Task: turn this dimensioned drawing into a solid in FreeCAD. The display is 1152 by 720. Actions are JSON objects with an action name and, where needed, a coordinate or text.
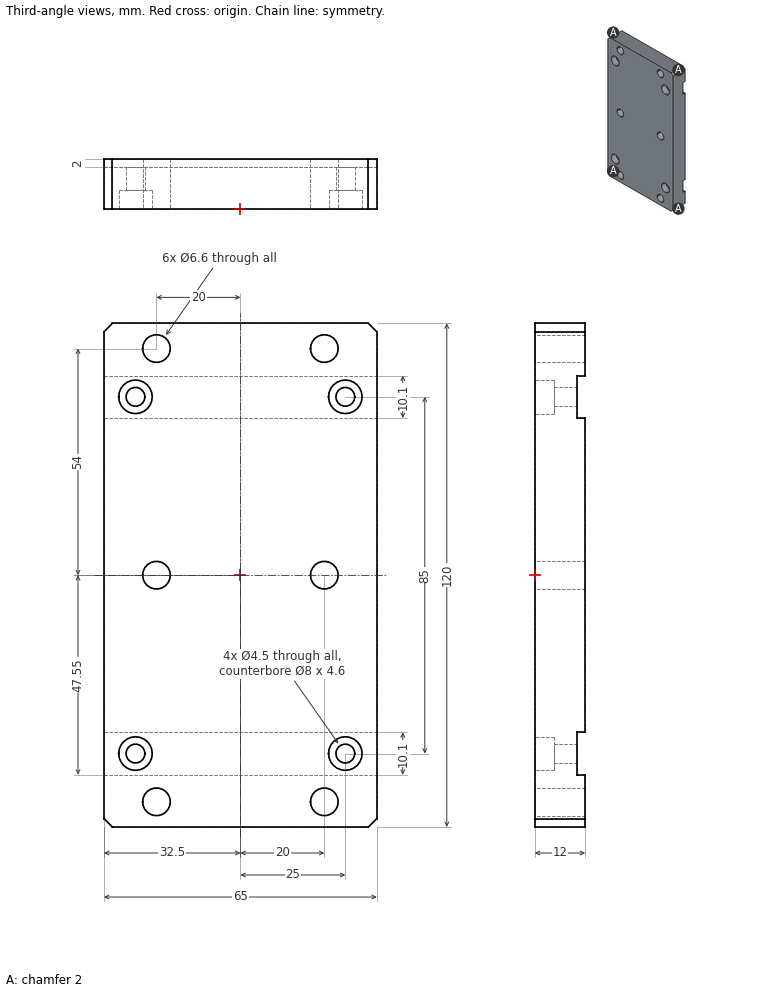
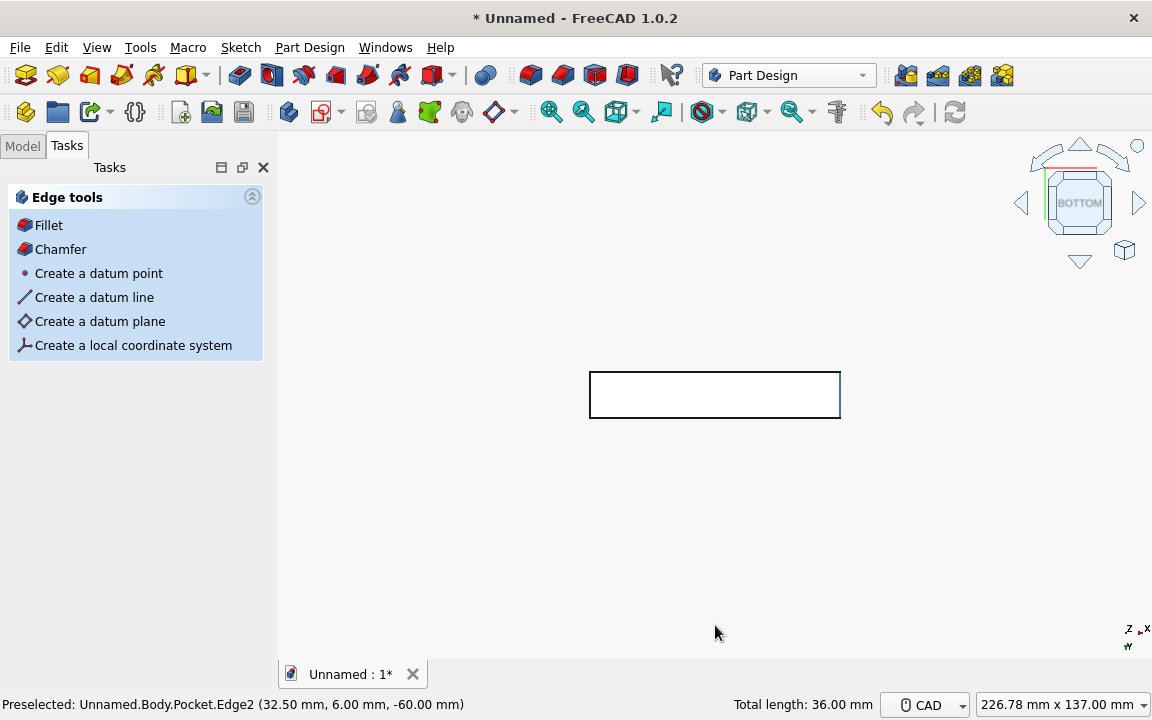
{"action": "key", "text": "v f"}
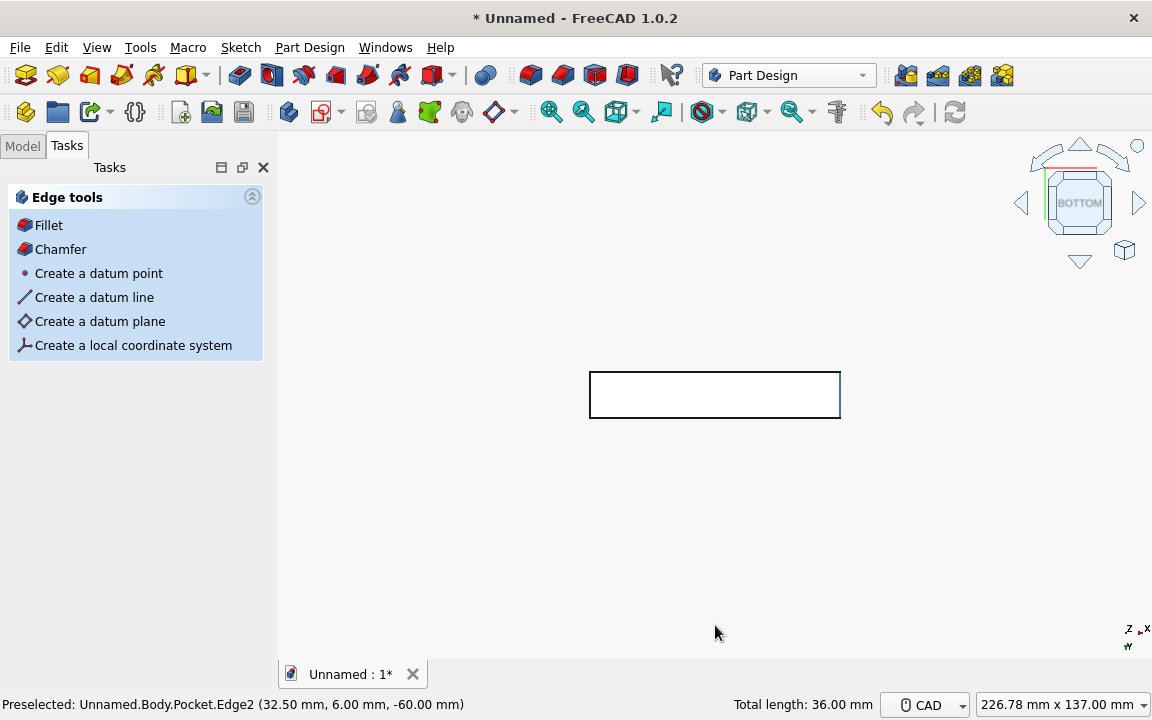
{"action": "left_click", "coordinate": [590, 394], "text": "ctrl"}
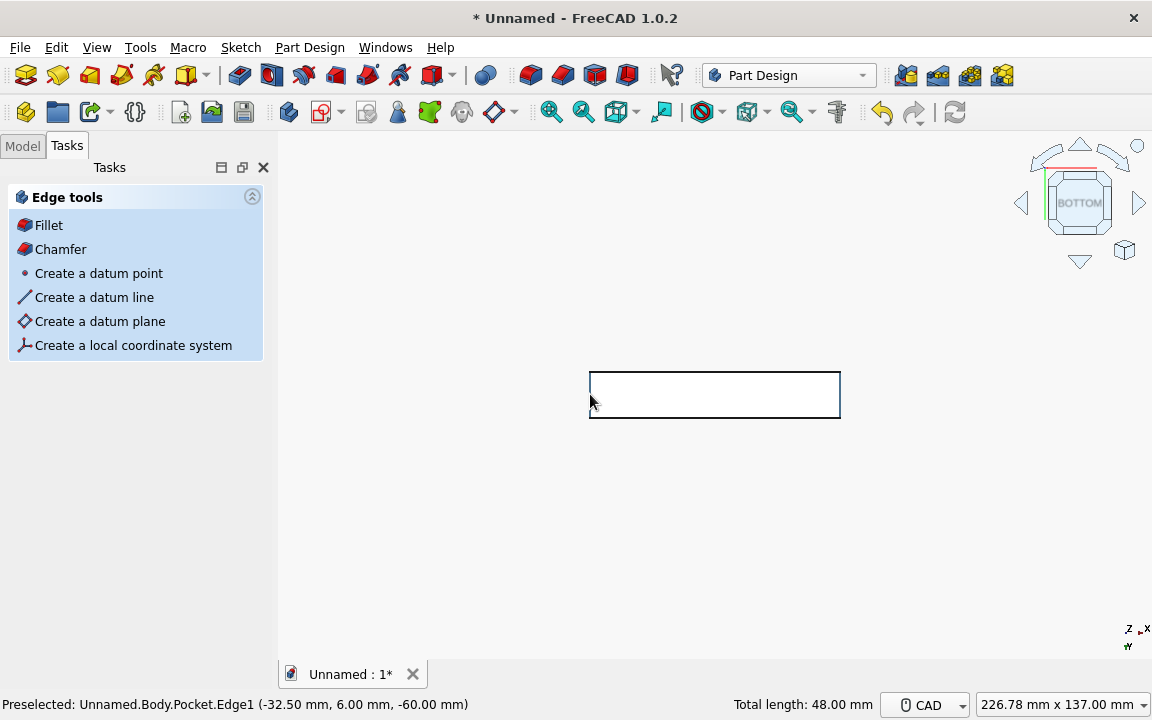
{"action": "left_click", "coordinate": [564, 76]}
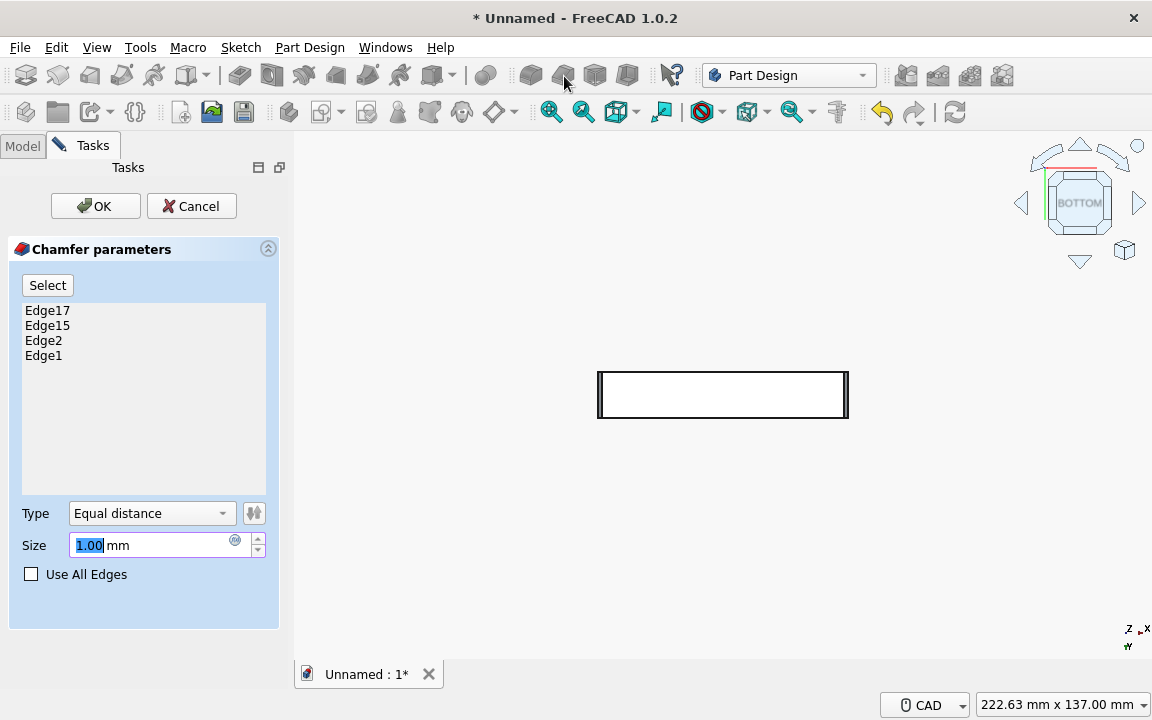
{"action": "type", "text": "2"}
{"action": "key", "text": "Tab"}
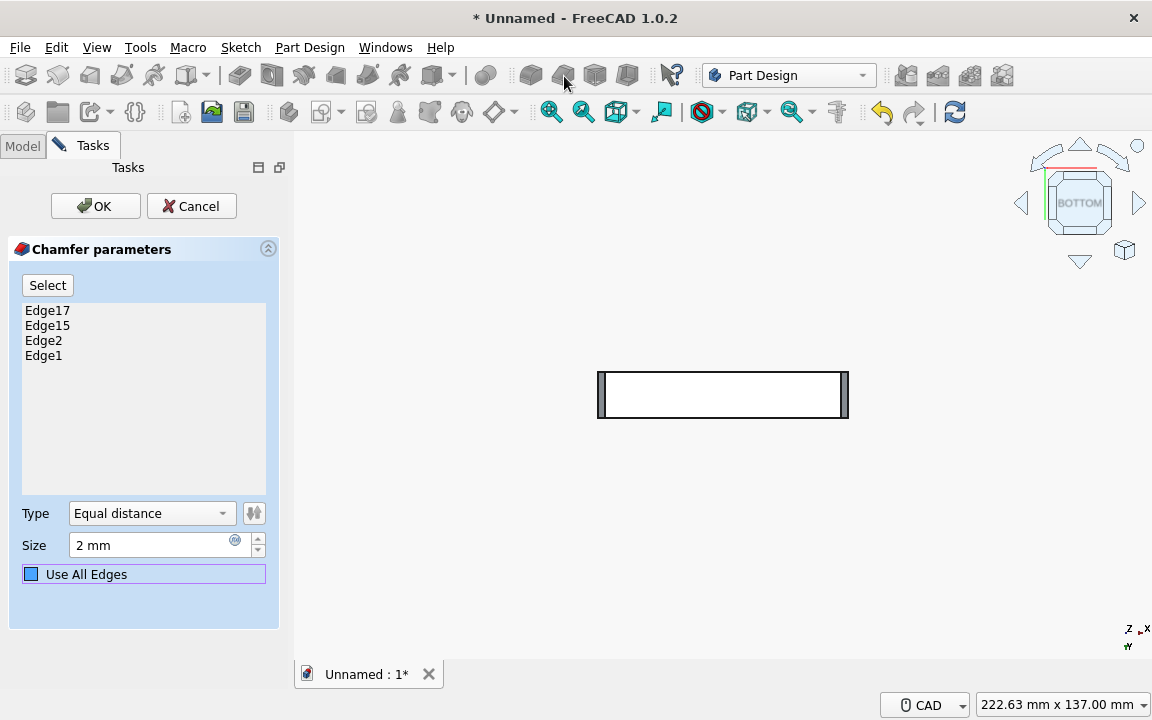
{"action": "left_click", "coordinate": [96, 206]}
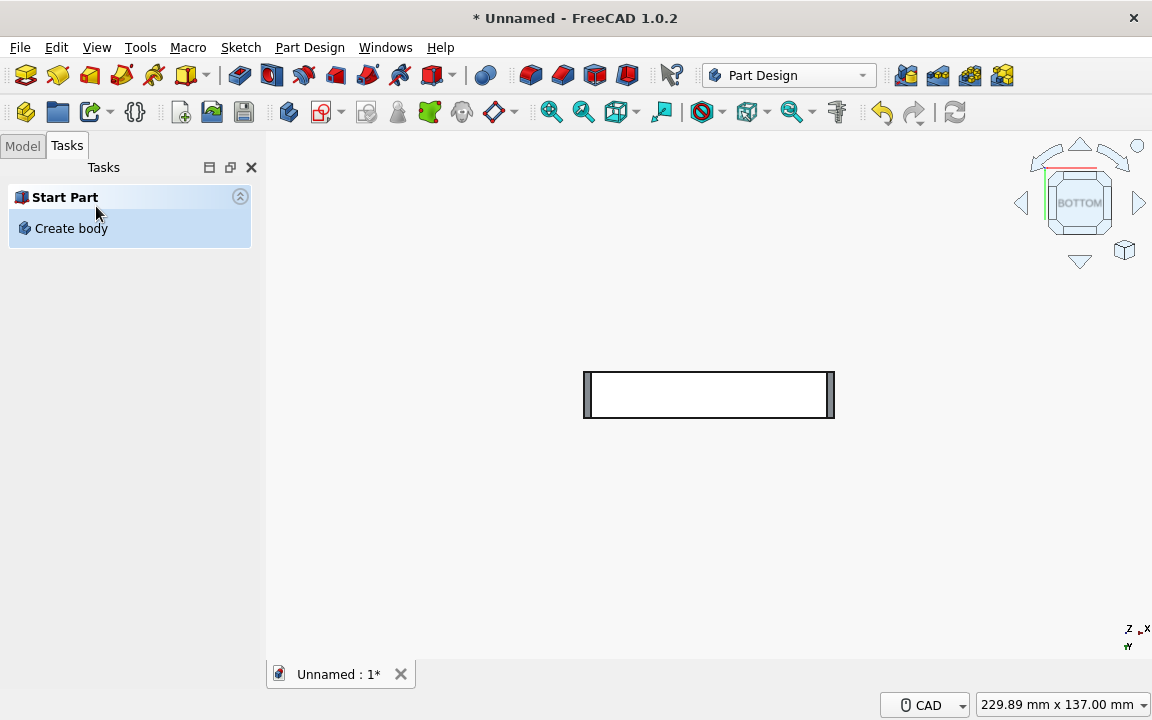
{"action": "key", "text": "v f"}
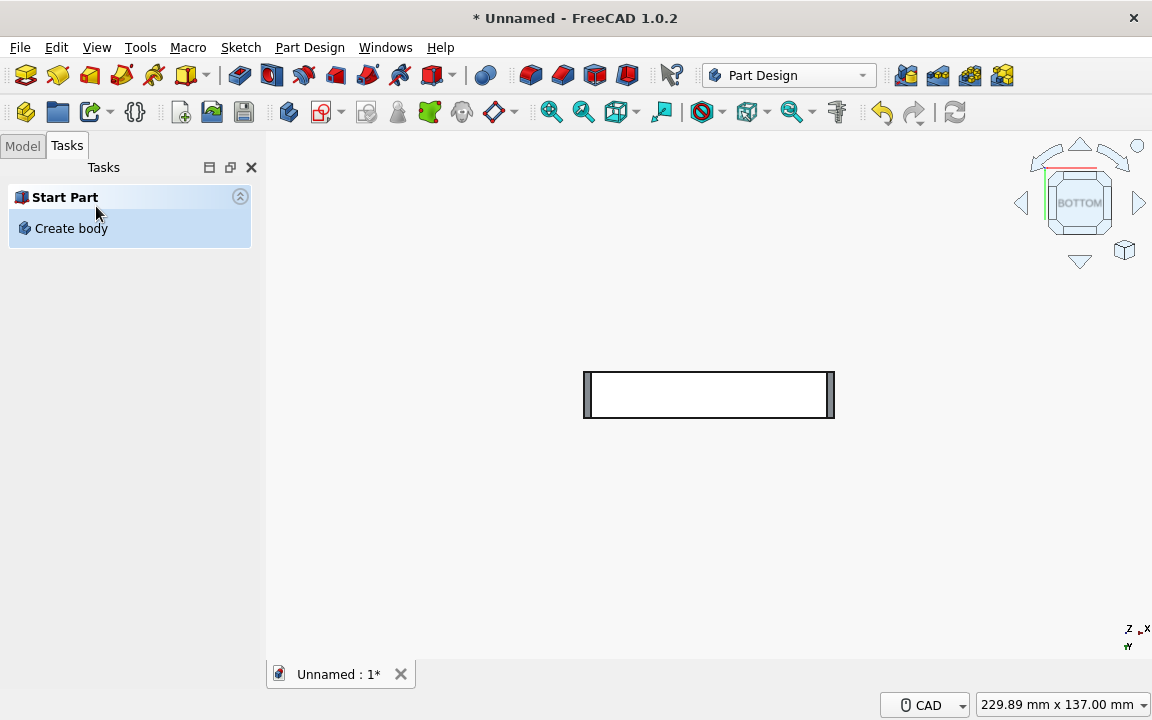
{"action": "key", "text": "0"}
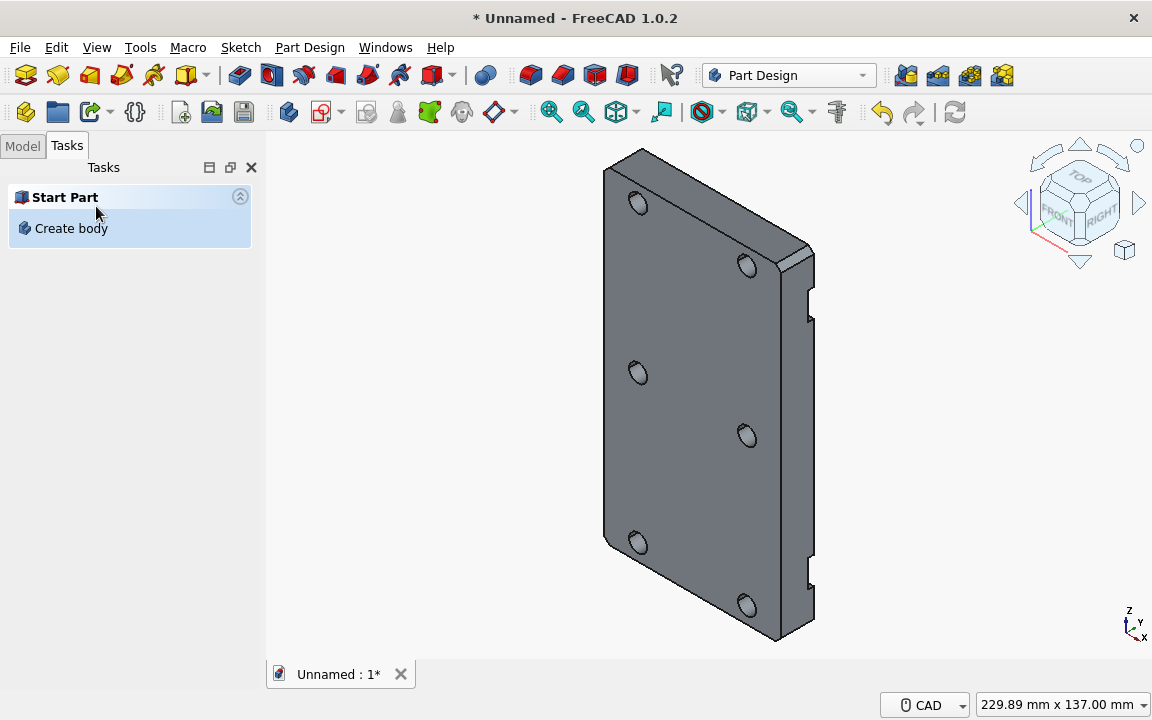
{"action": "left_click", "coordinate": [693, 296]}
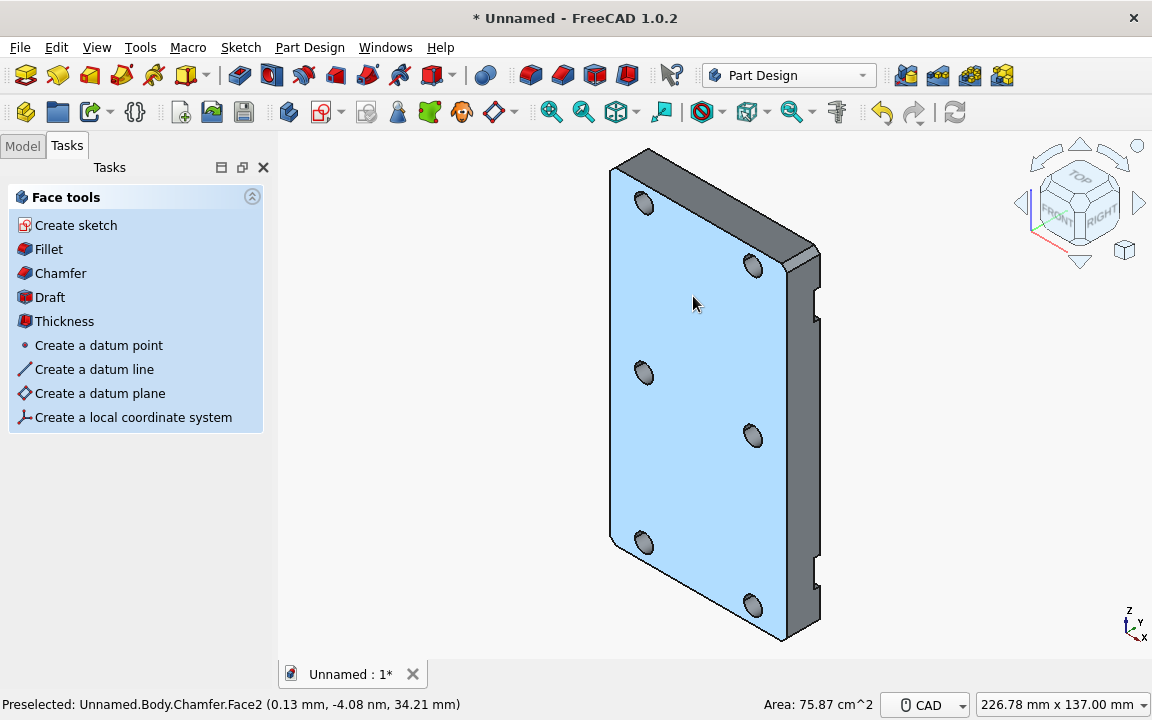
{"action": "left_click", "coordinate": [322, 112]}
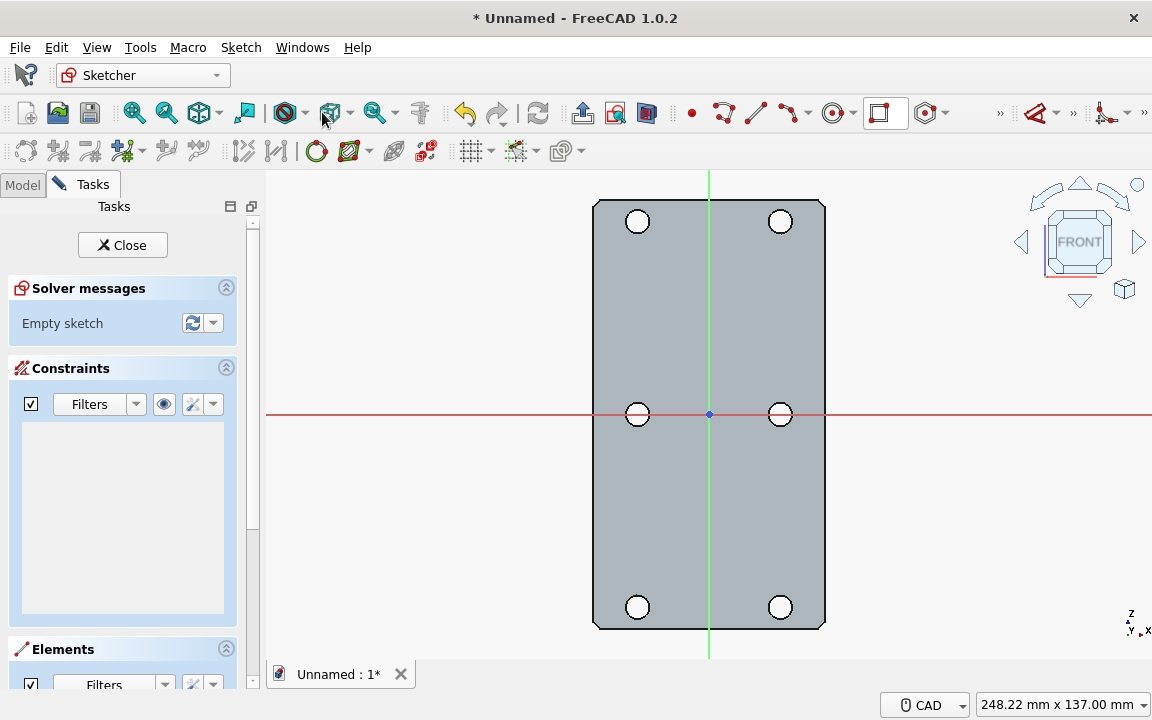
{"action": "left_click", "coordinate": [834, 114]}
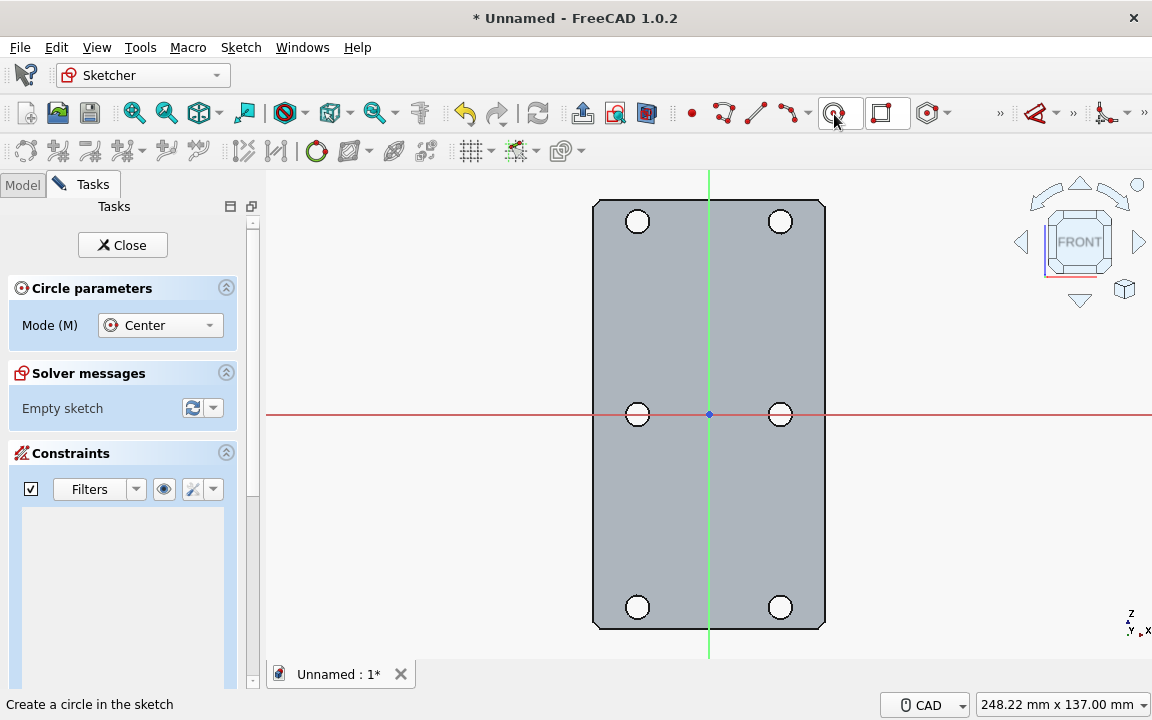
{"action": "scroll", "coordinate": [798, 566], "scroll_direction": "up", "scroll_amount": 6}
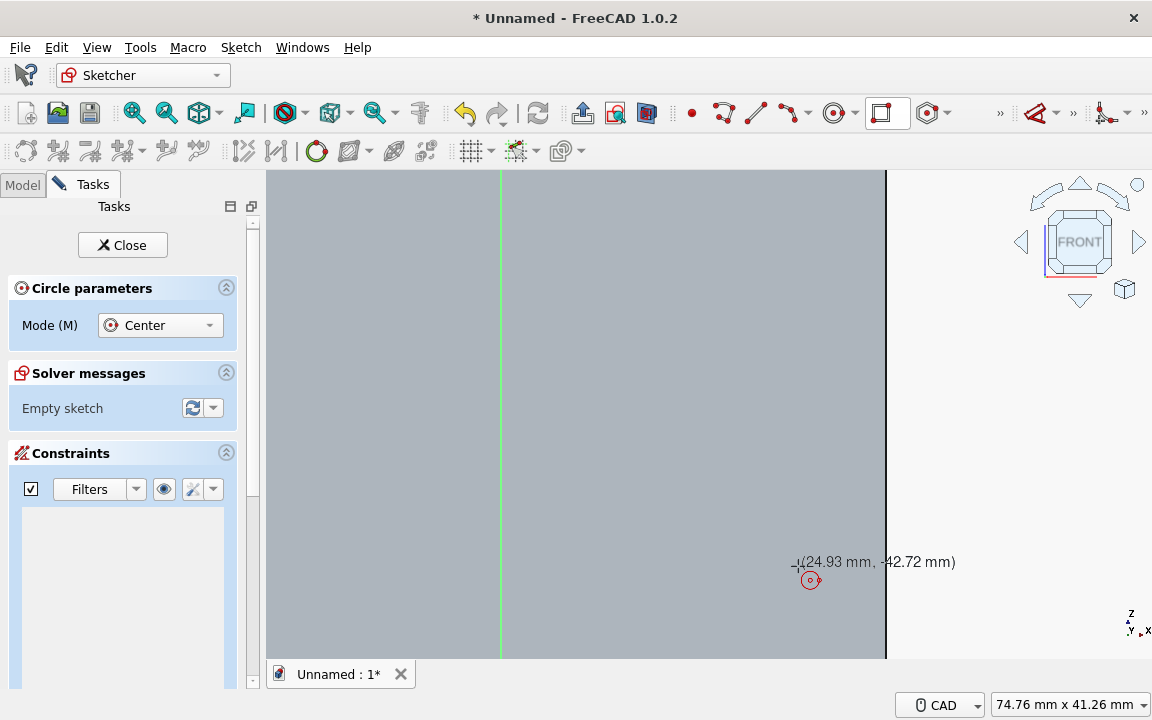
{"action": "left_click", "coordinate": [797, 565]}
{"action": "mouse_move", "coordinate": [816, 546]}